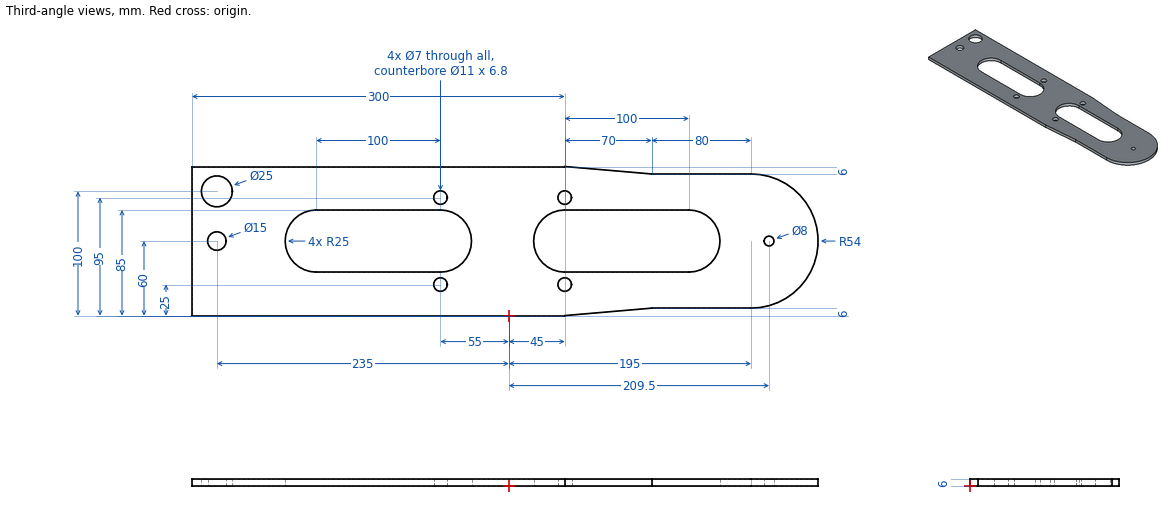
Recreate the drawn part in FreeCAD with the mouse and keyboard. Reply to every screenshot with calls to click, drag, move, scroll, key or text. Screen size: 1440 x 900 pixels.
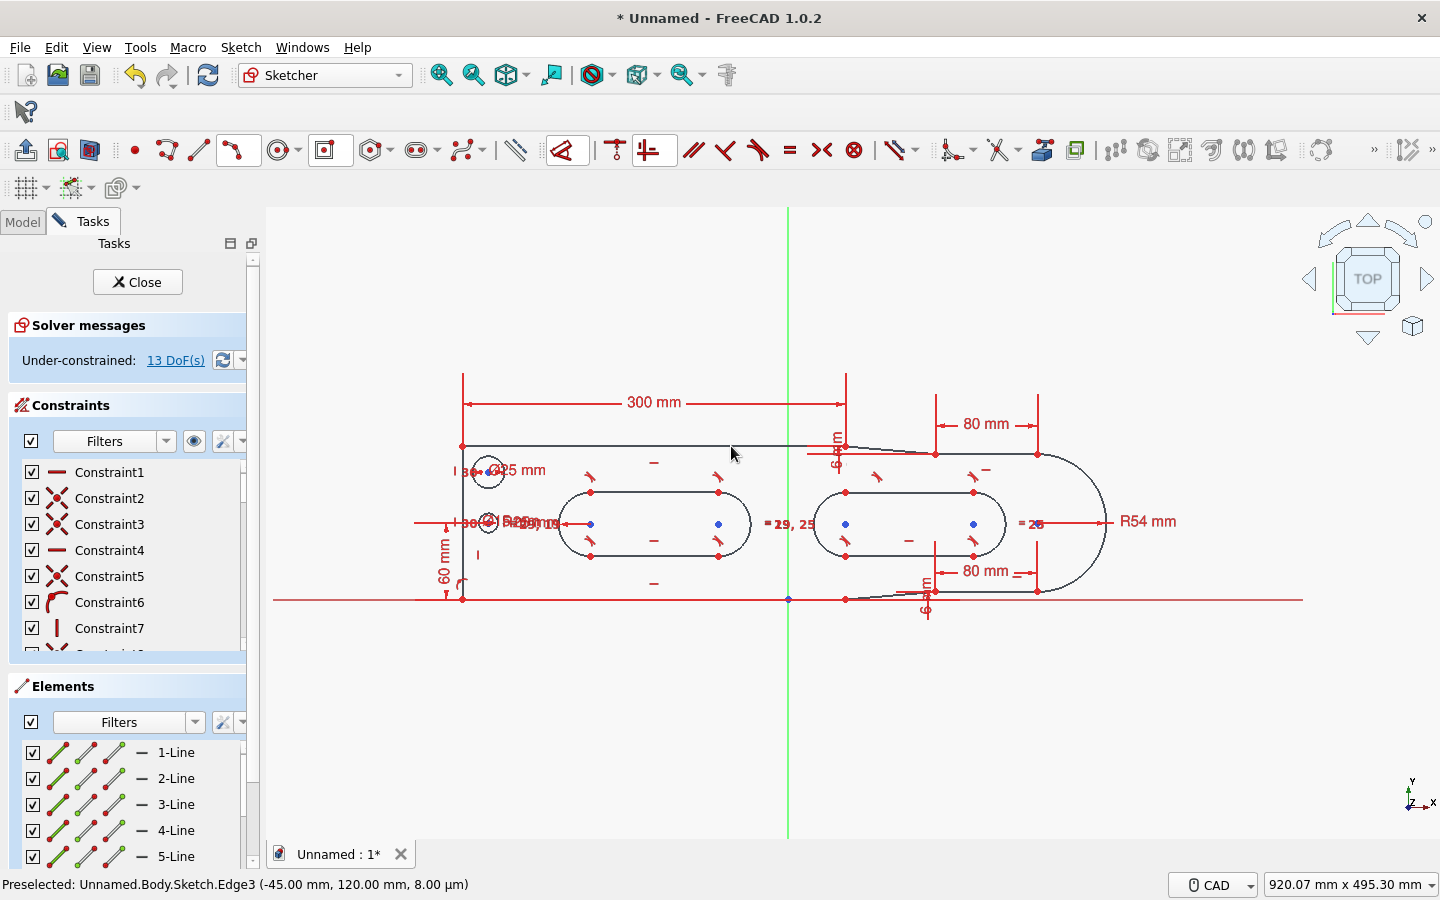
click(578, 600)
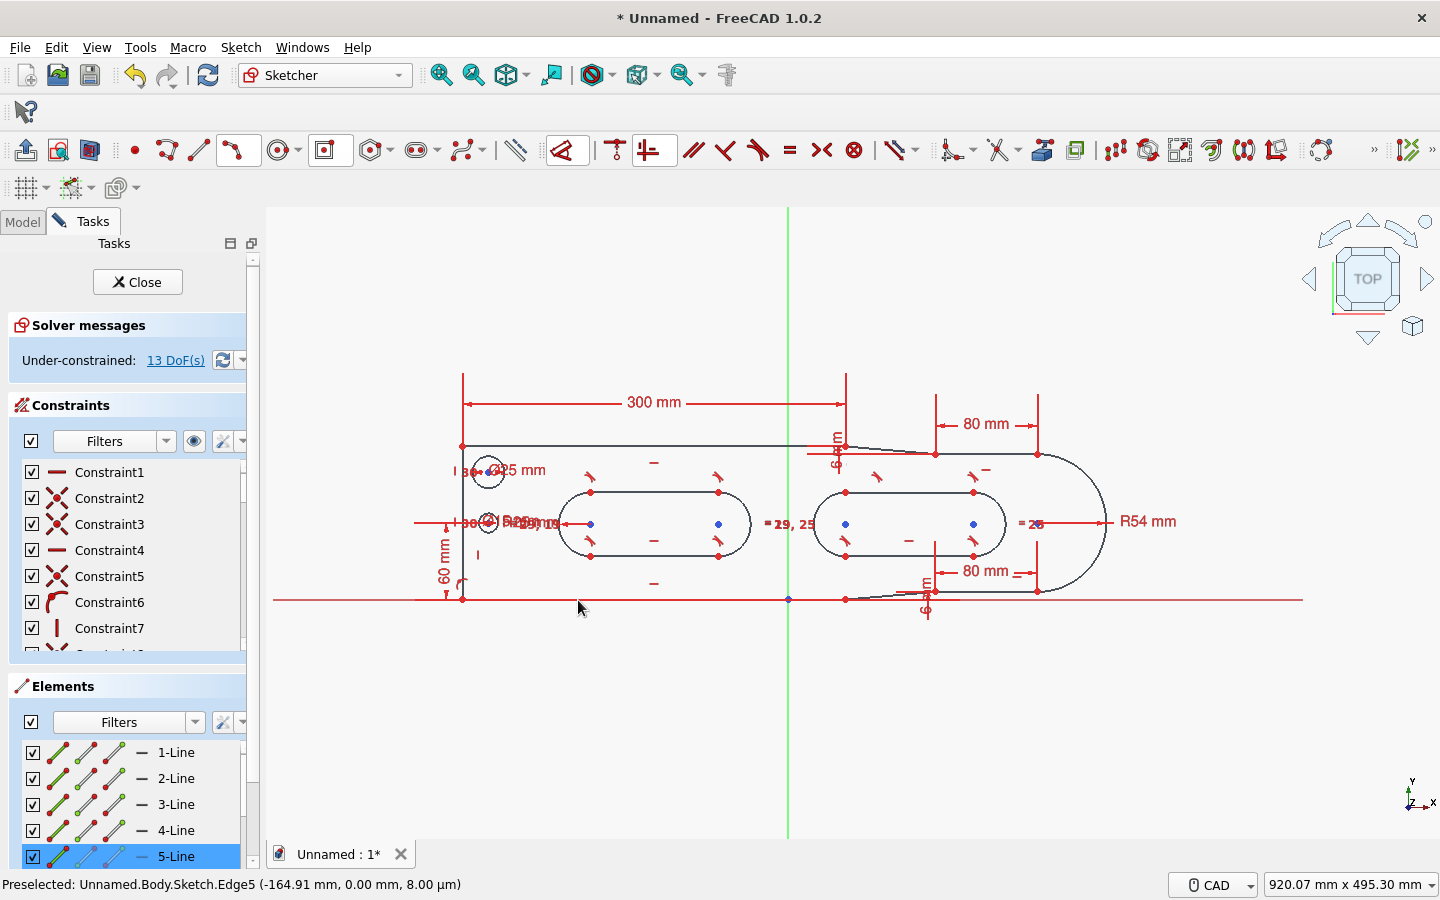
key(l)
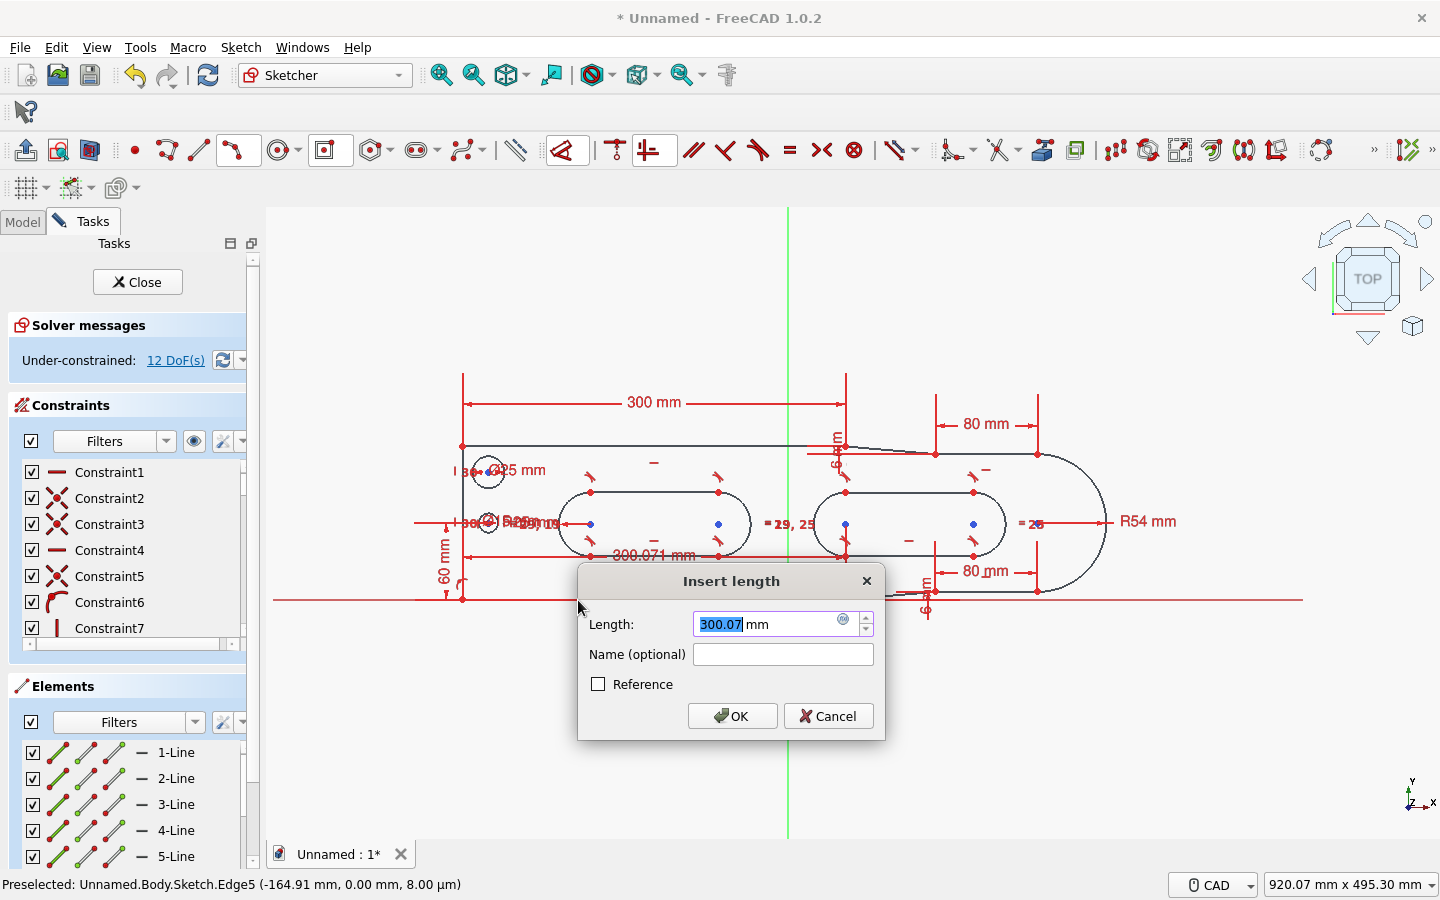
text(300)
key(Return)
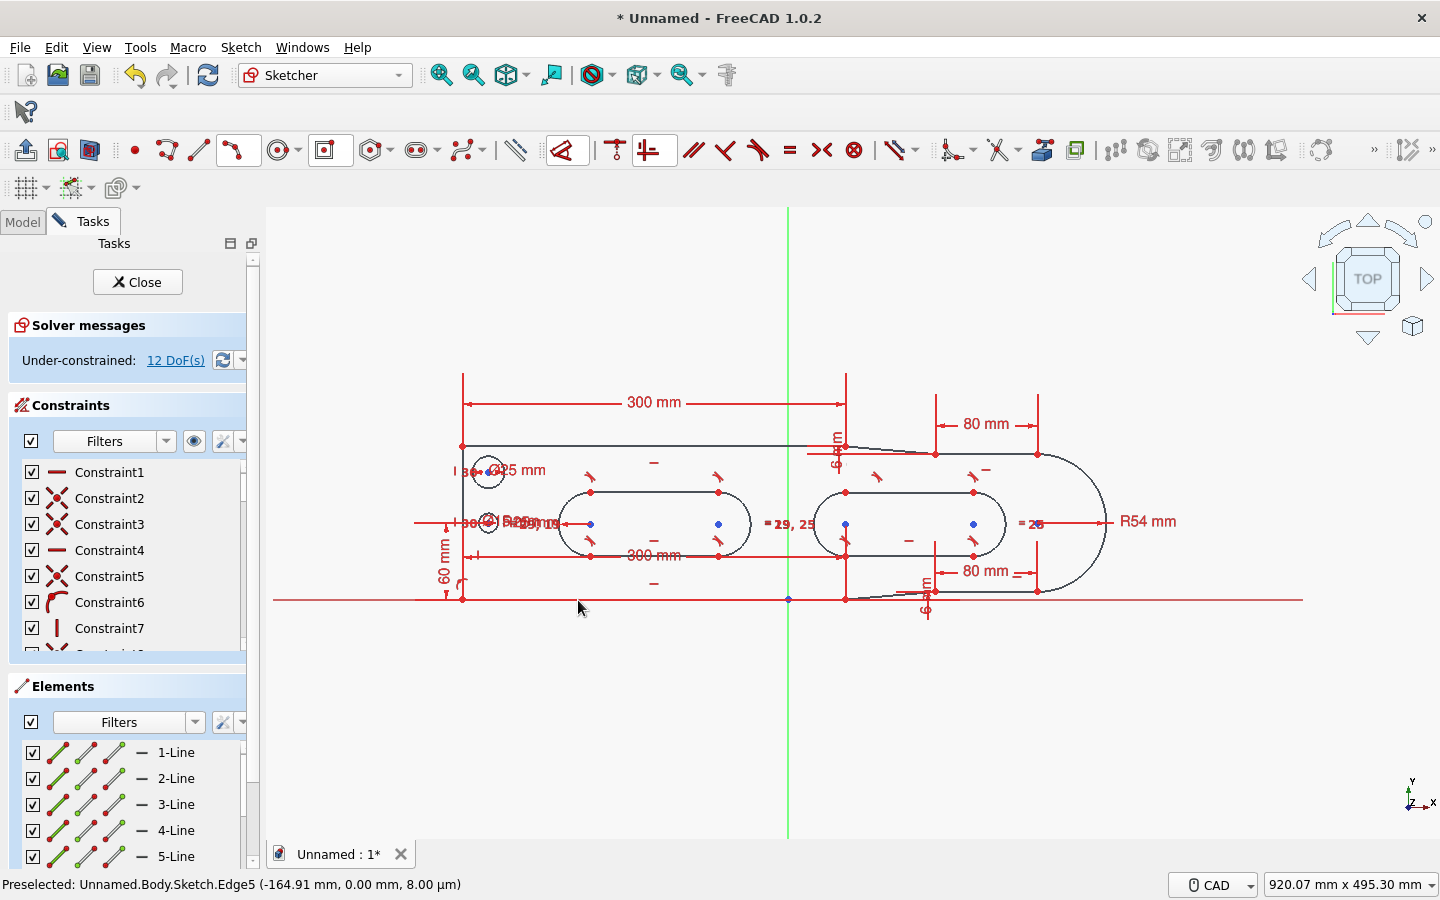
click(629, 492)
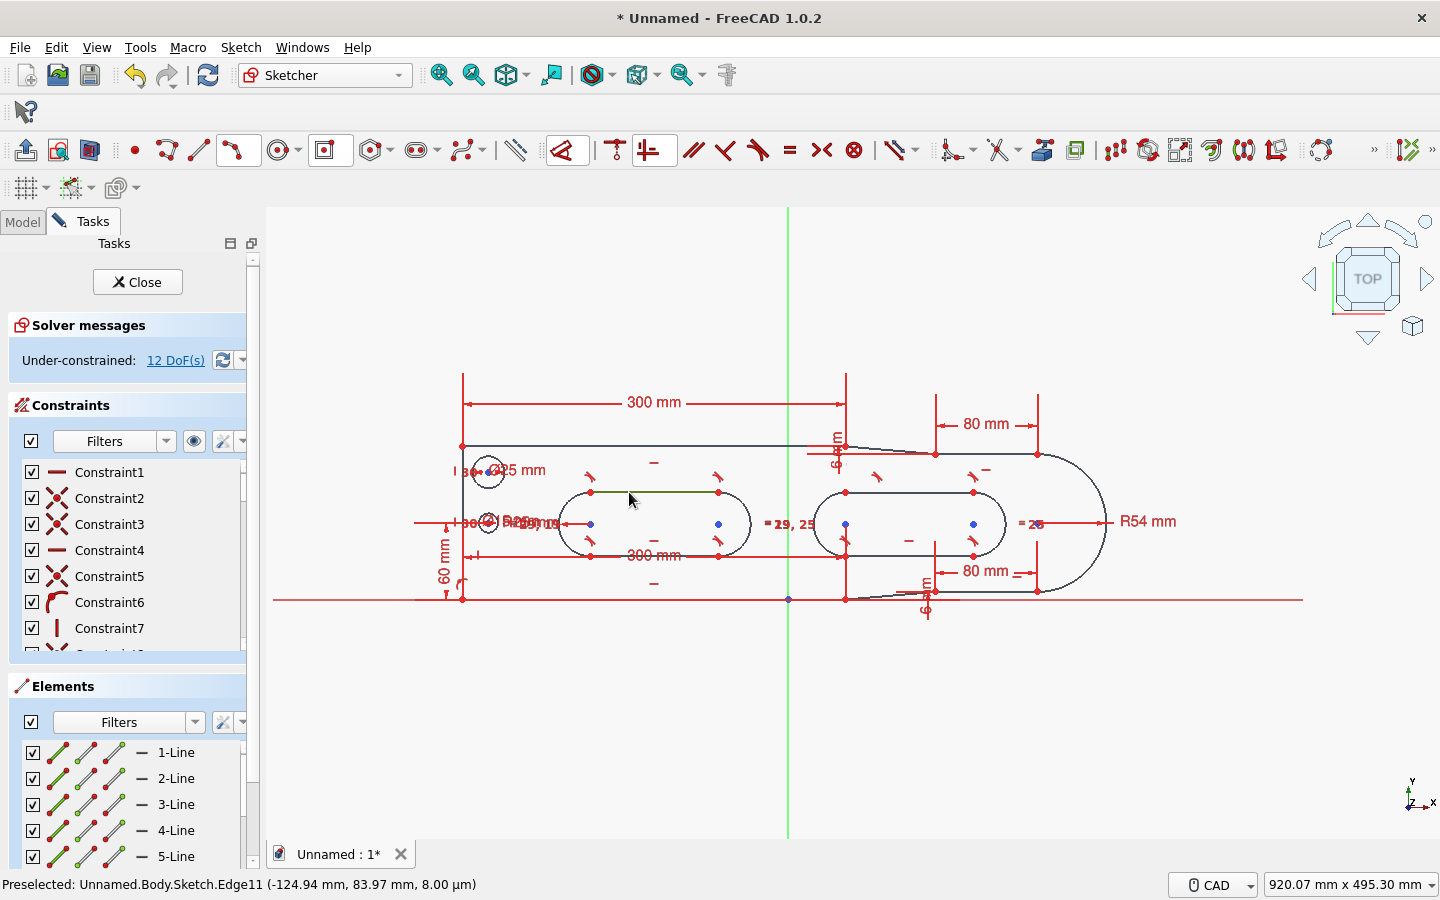
key(l)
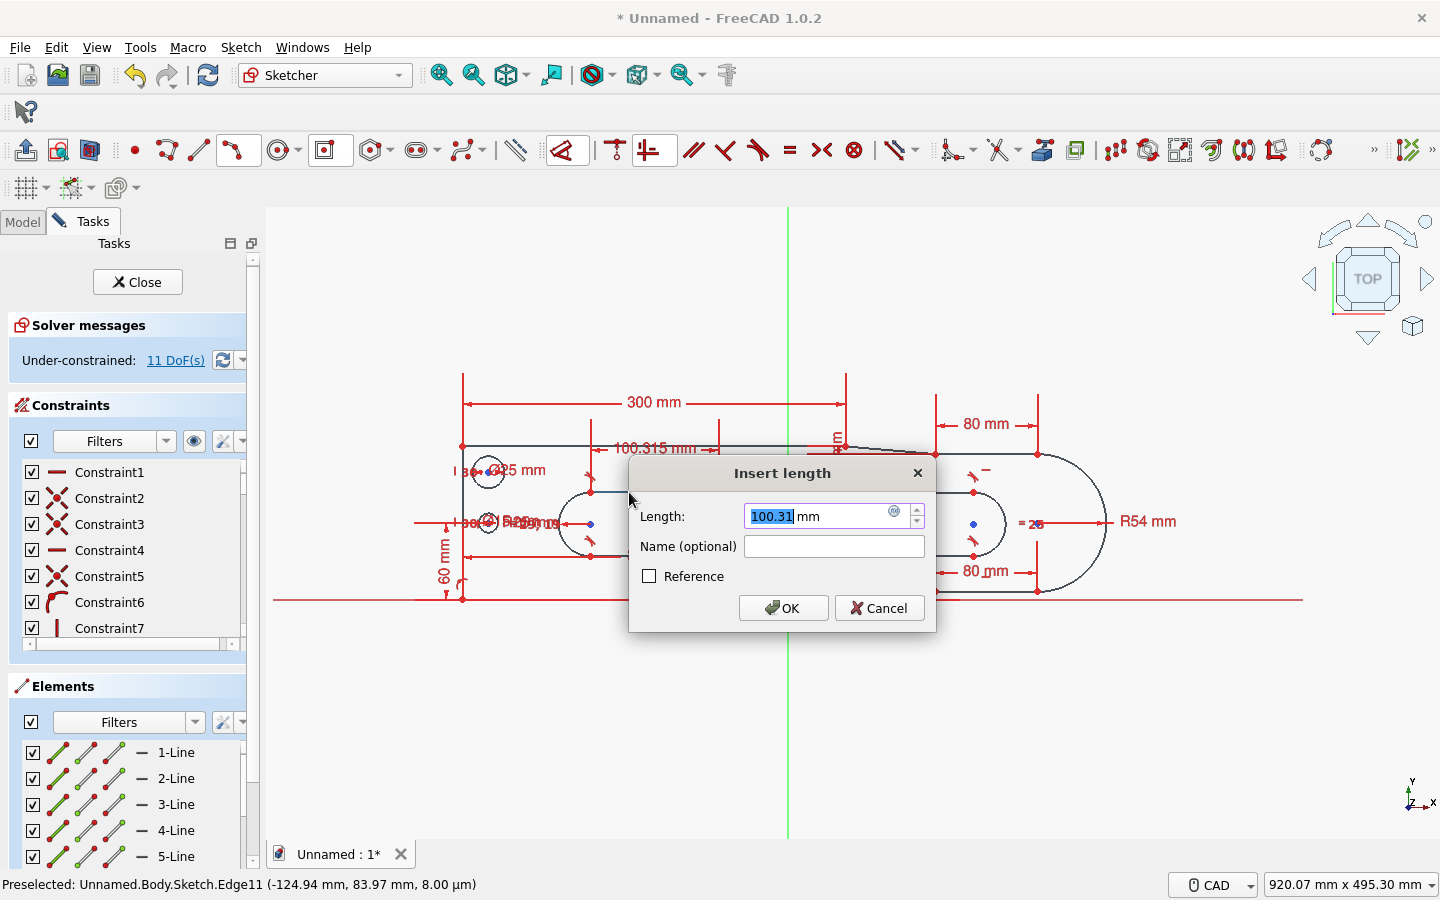
text(100)
key(Return)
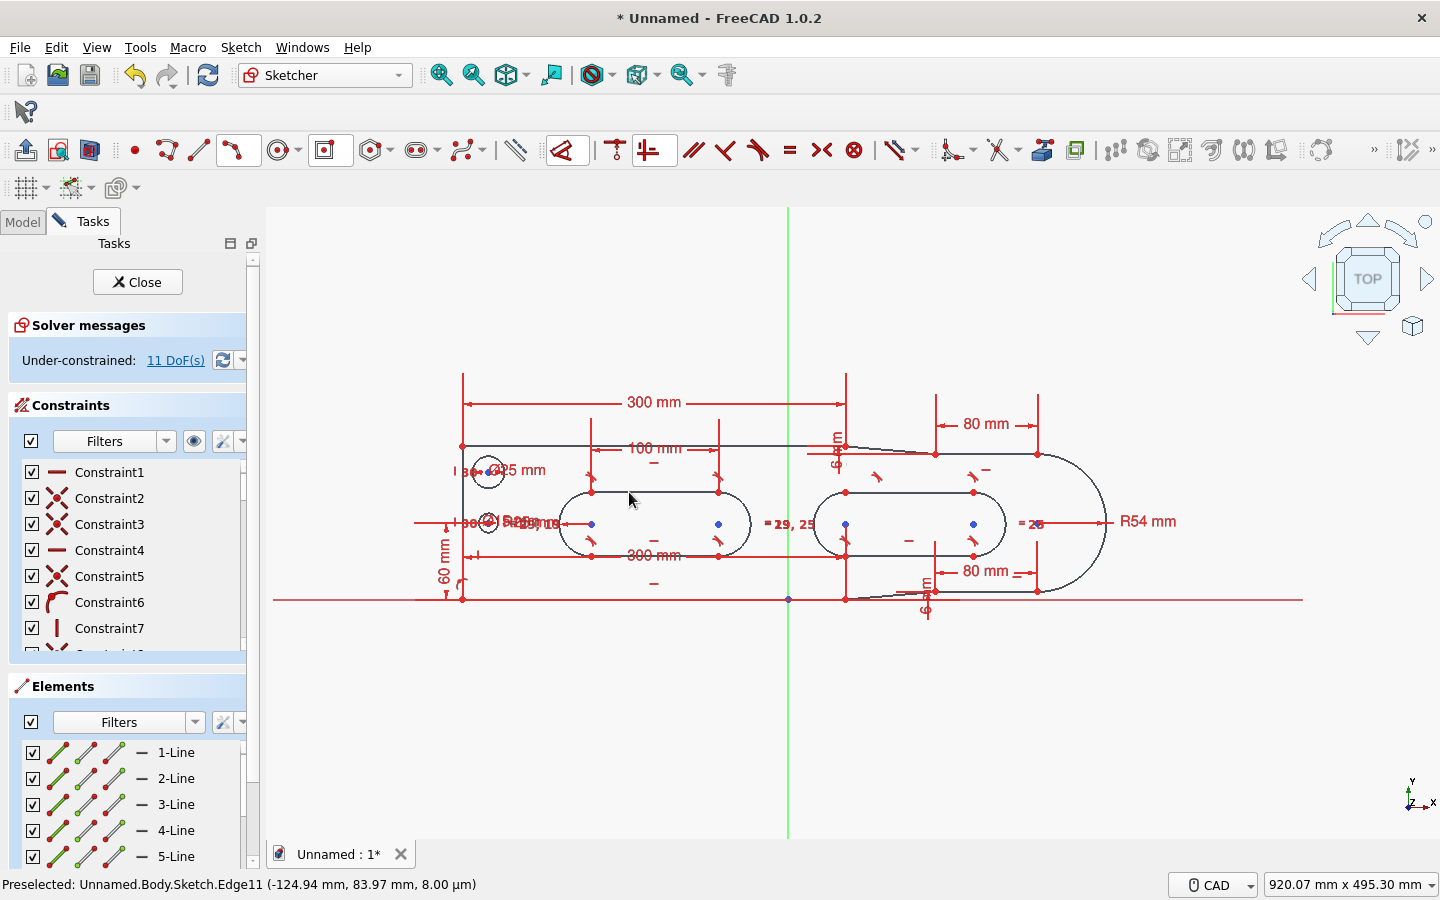
click(884, 493)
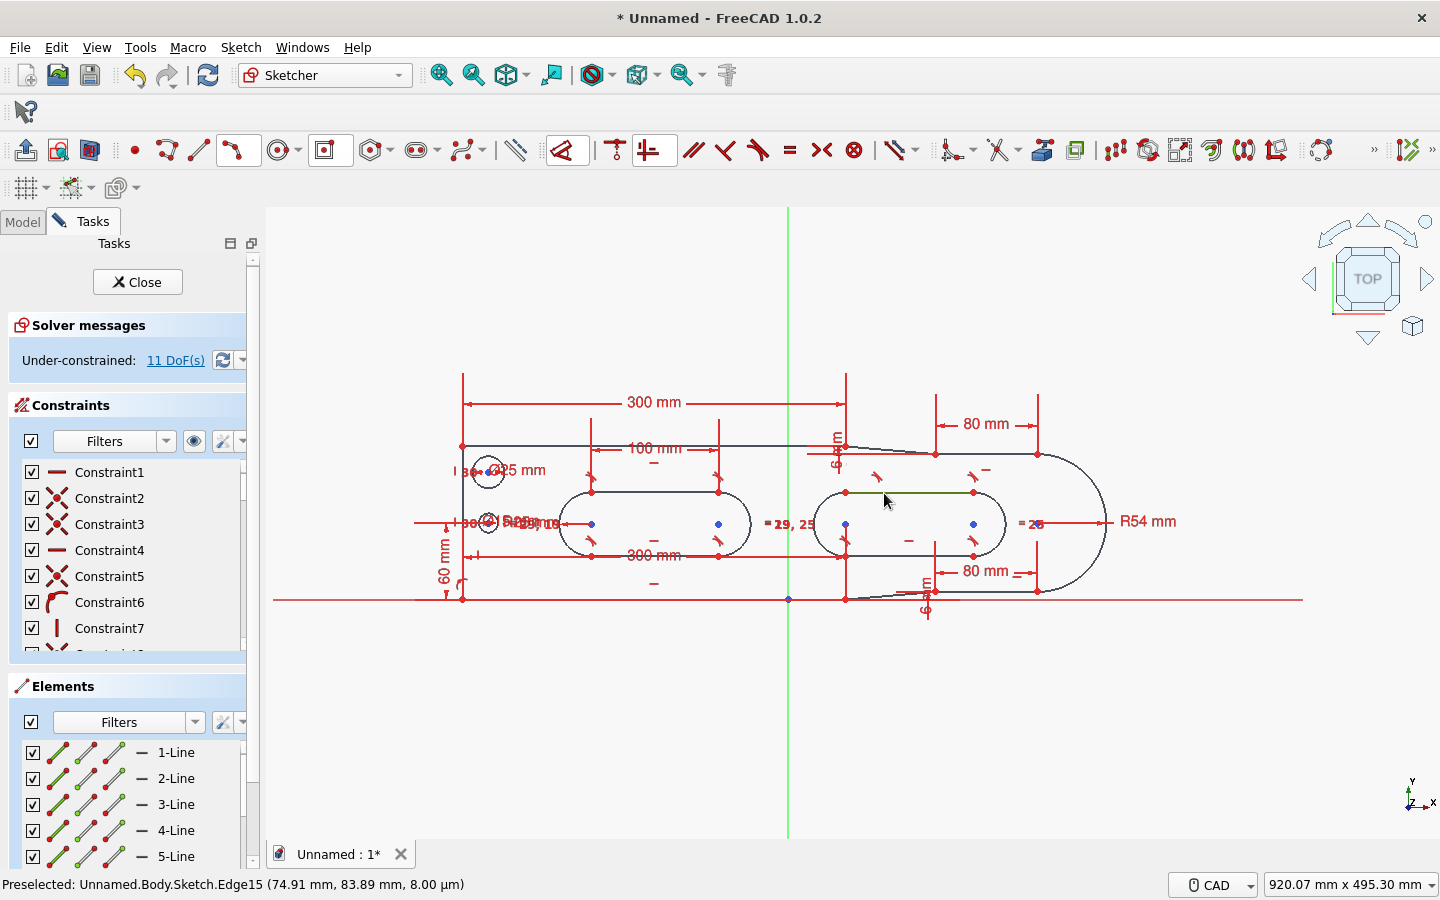
click(584, 150)